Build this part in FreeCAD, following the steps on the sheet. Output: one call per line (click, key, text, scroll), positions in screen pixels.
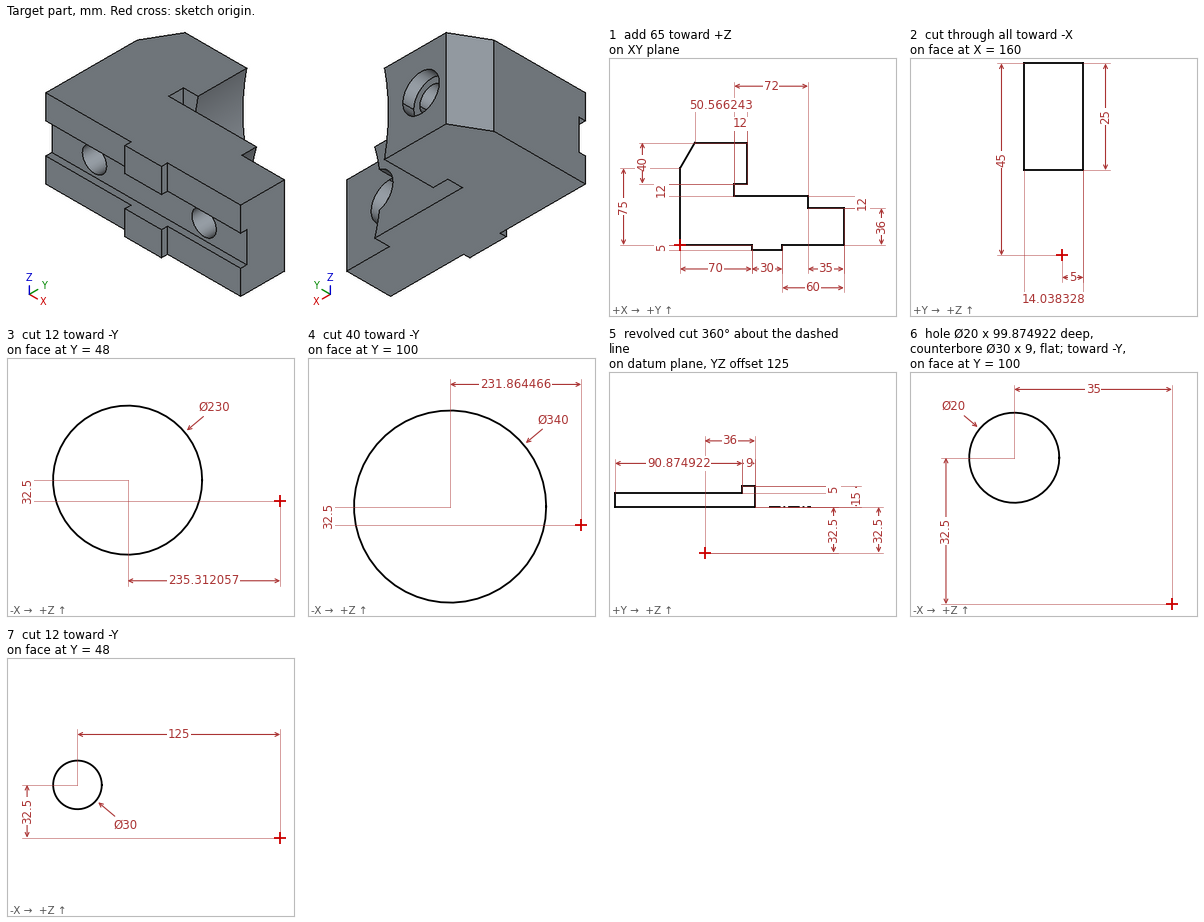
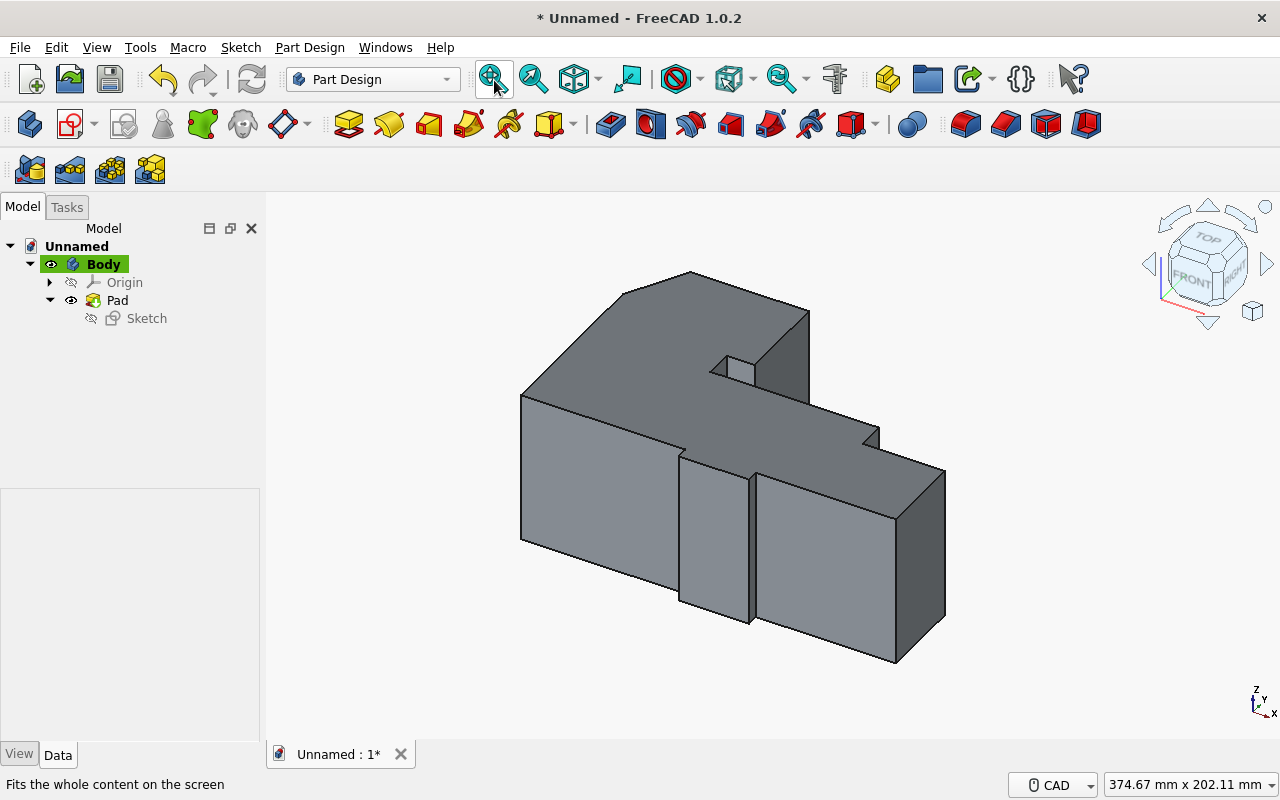
click(921, 546)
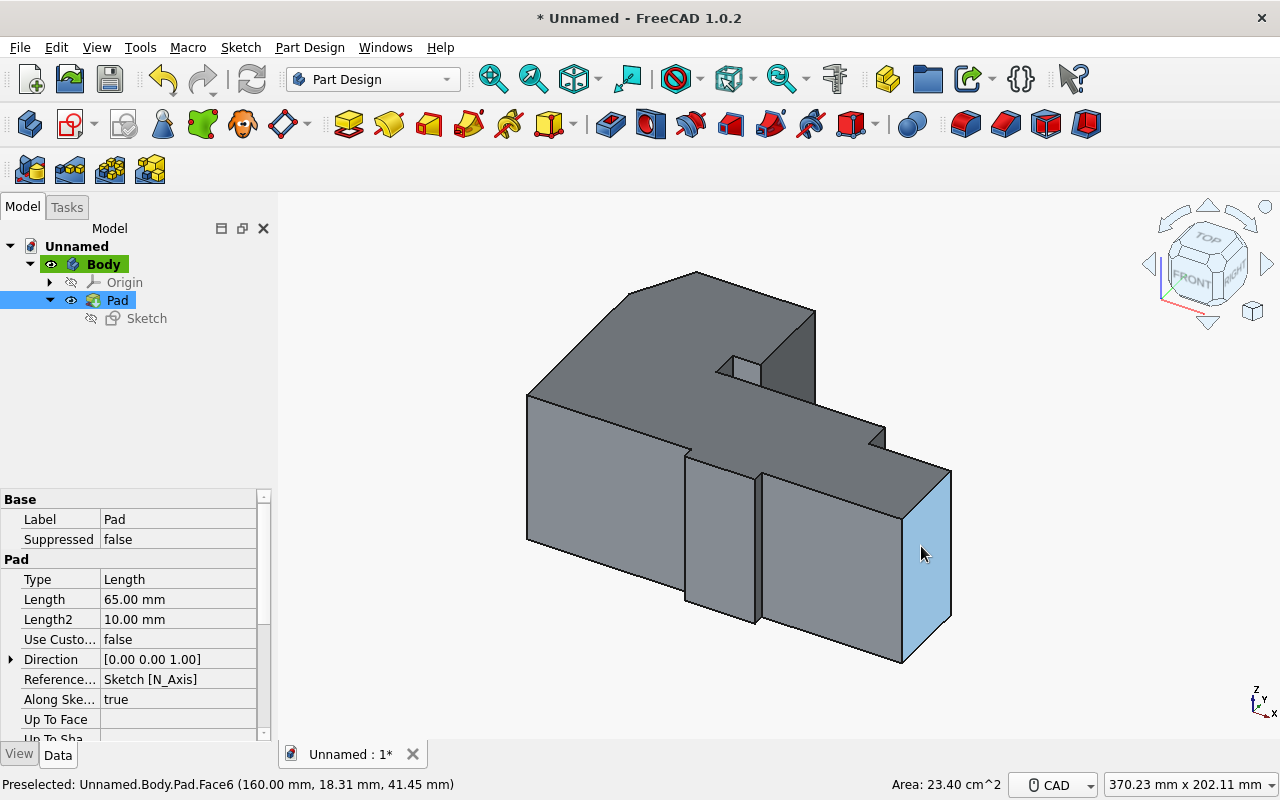
click(70, 124)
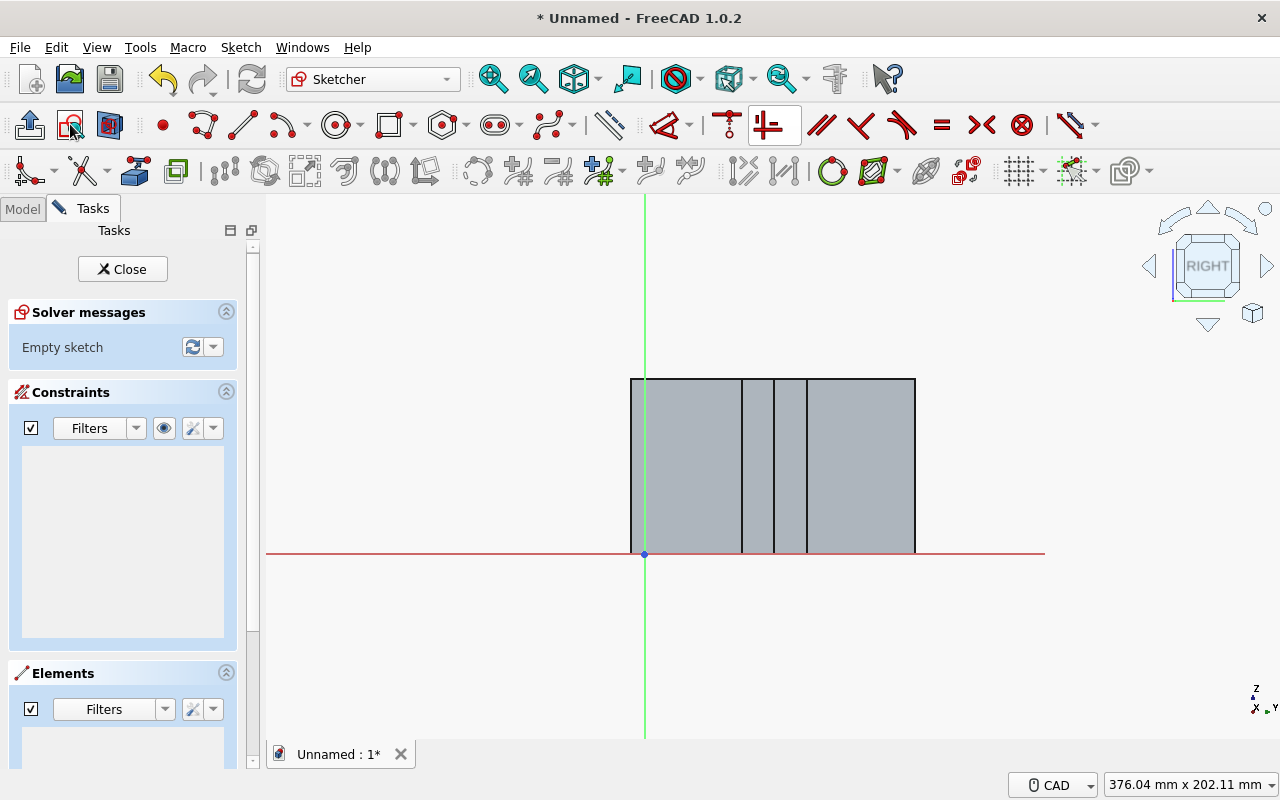
scroll(602, 509, up, 5)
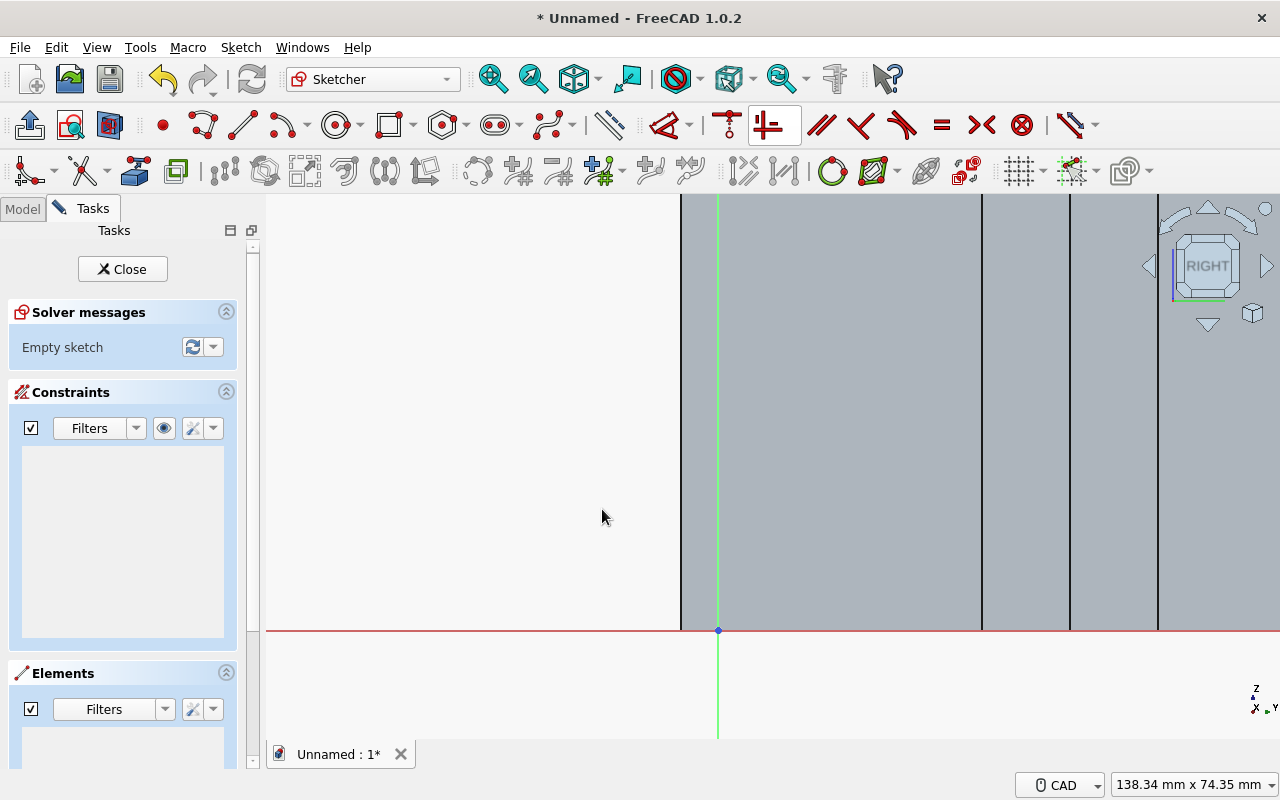
click(390, 126)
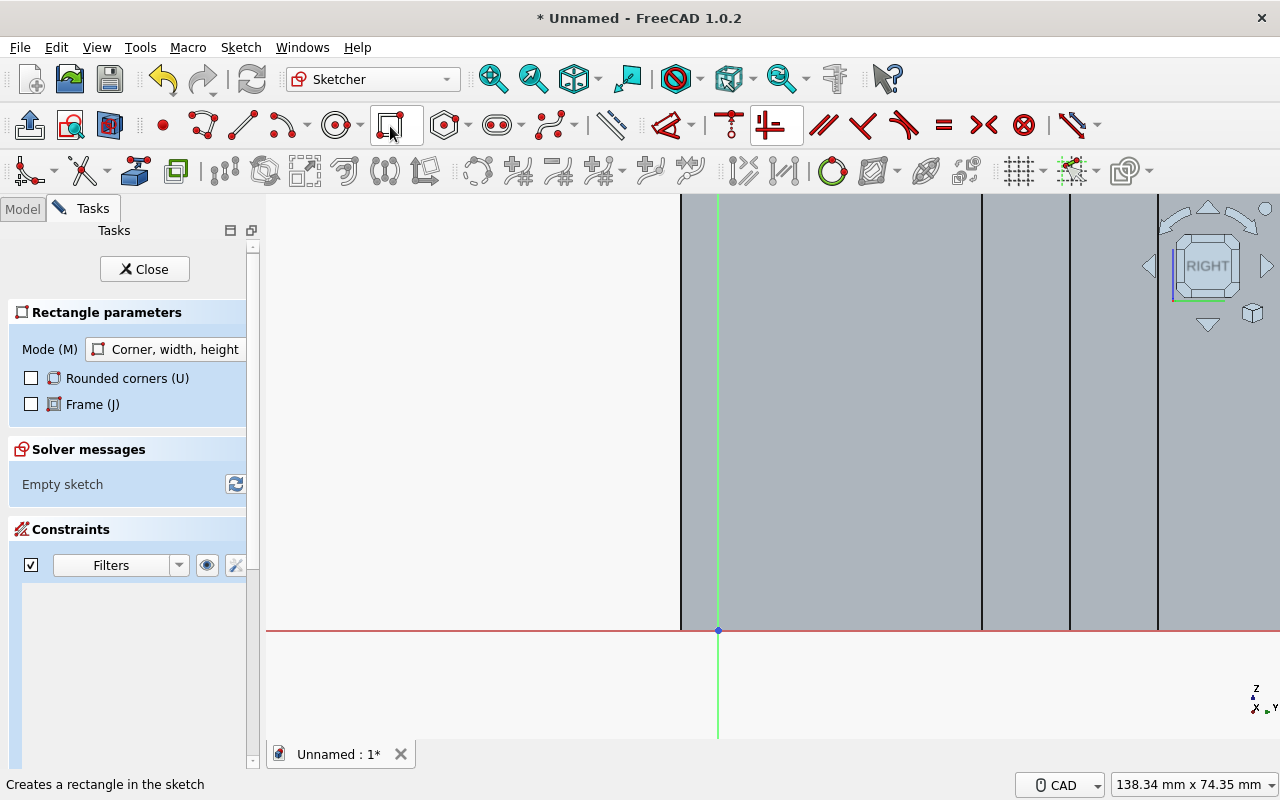
click(652, 301)
move(755, 484)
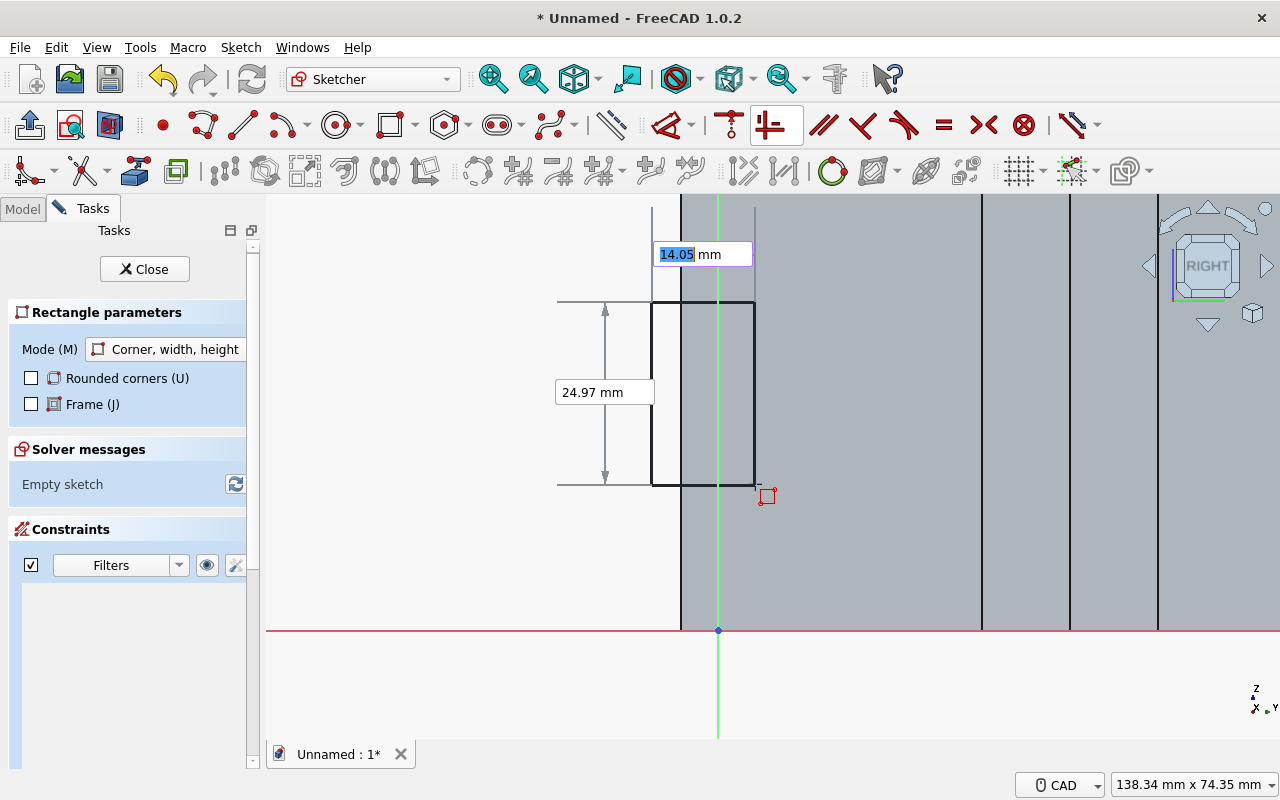
text(14.038328)
key(Tab)
text(25)
key(Return)
key(Escape)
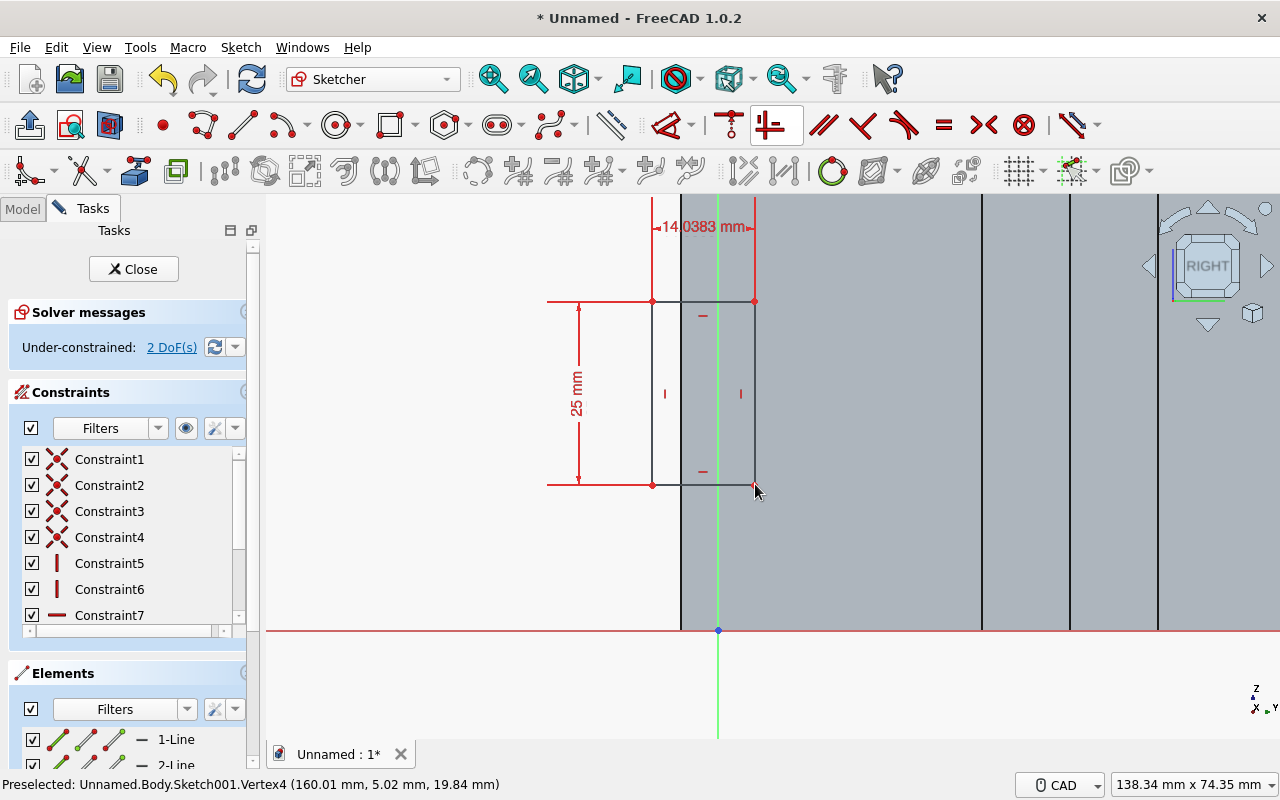
click(666, 126)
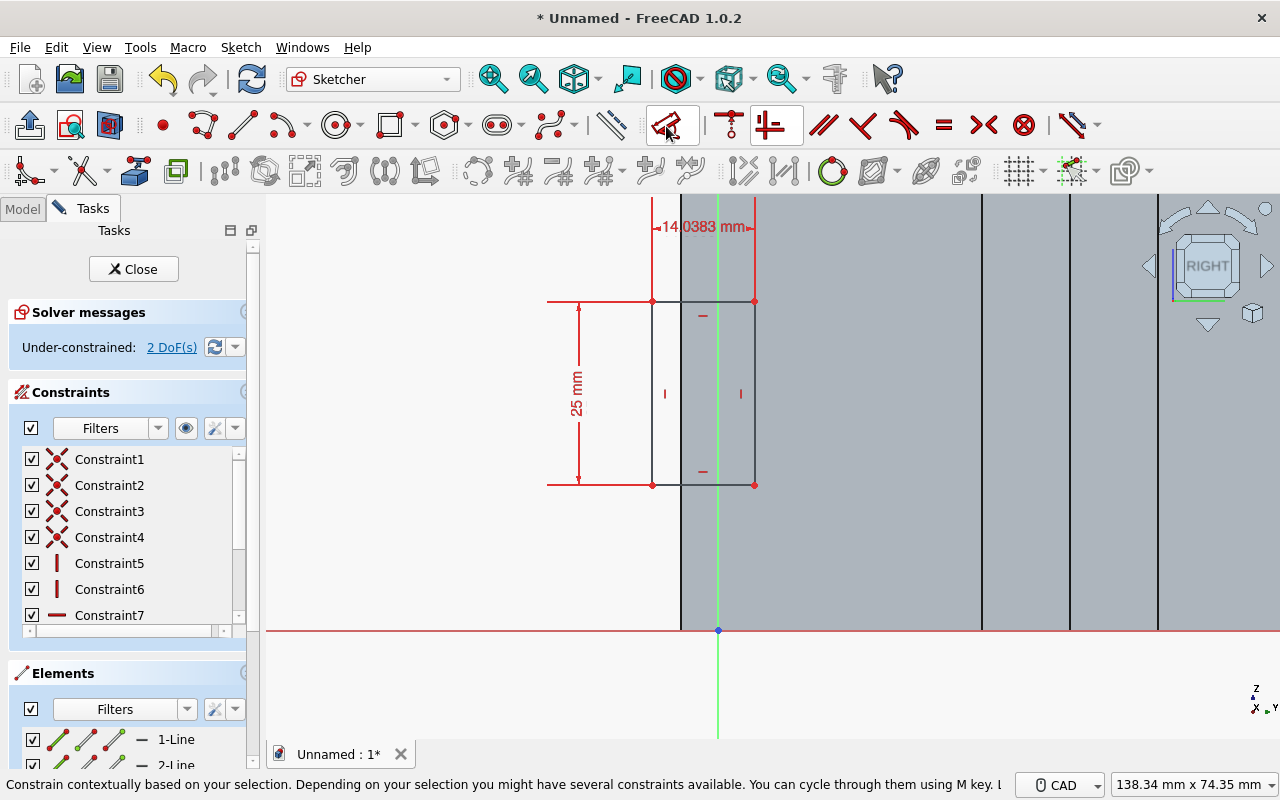
click(755, 485)
click(736, 665)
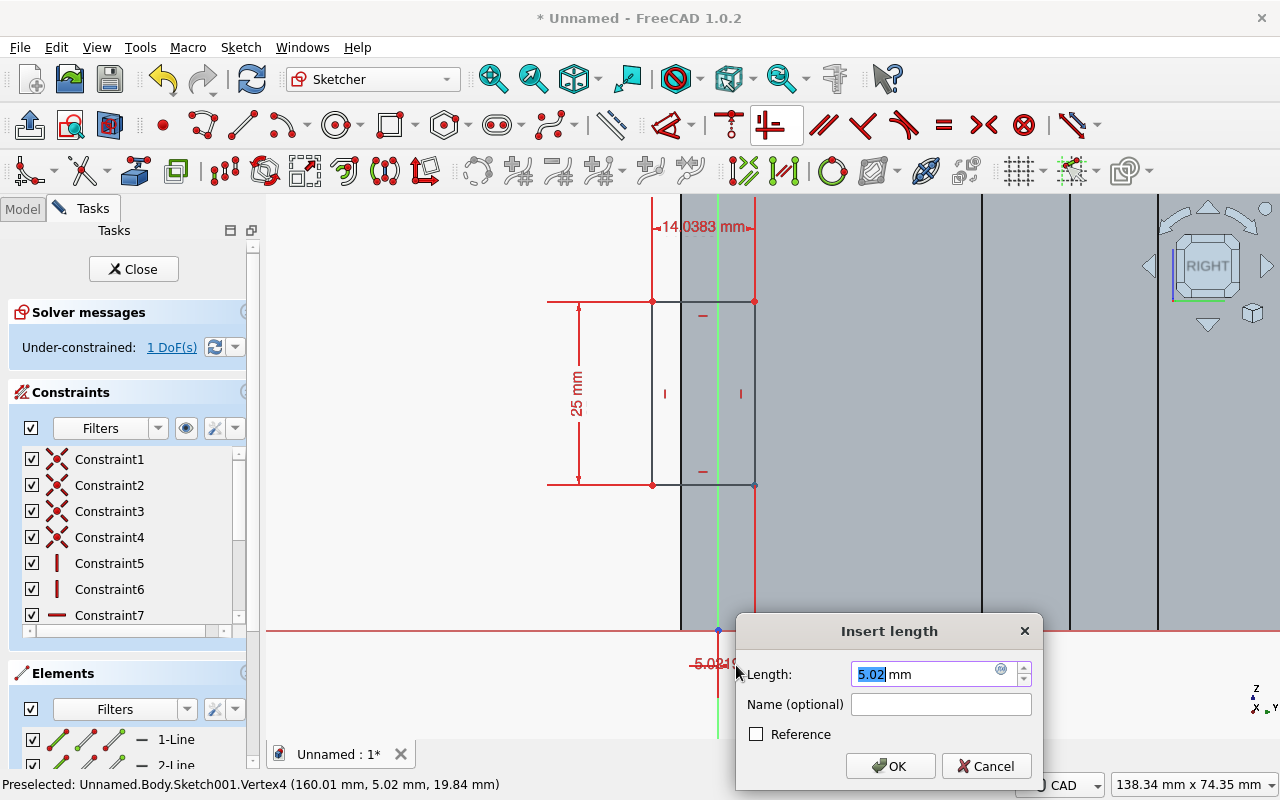
text(5)
key(Return)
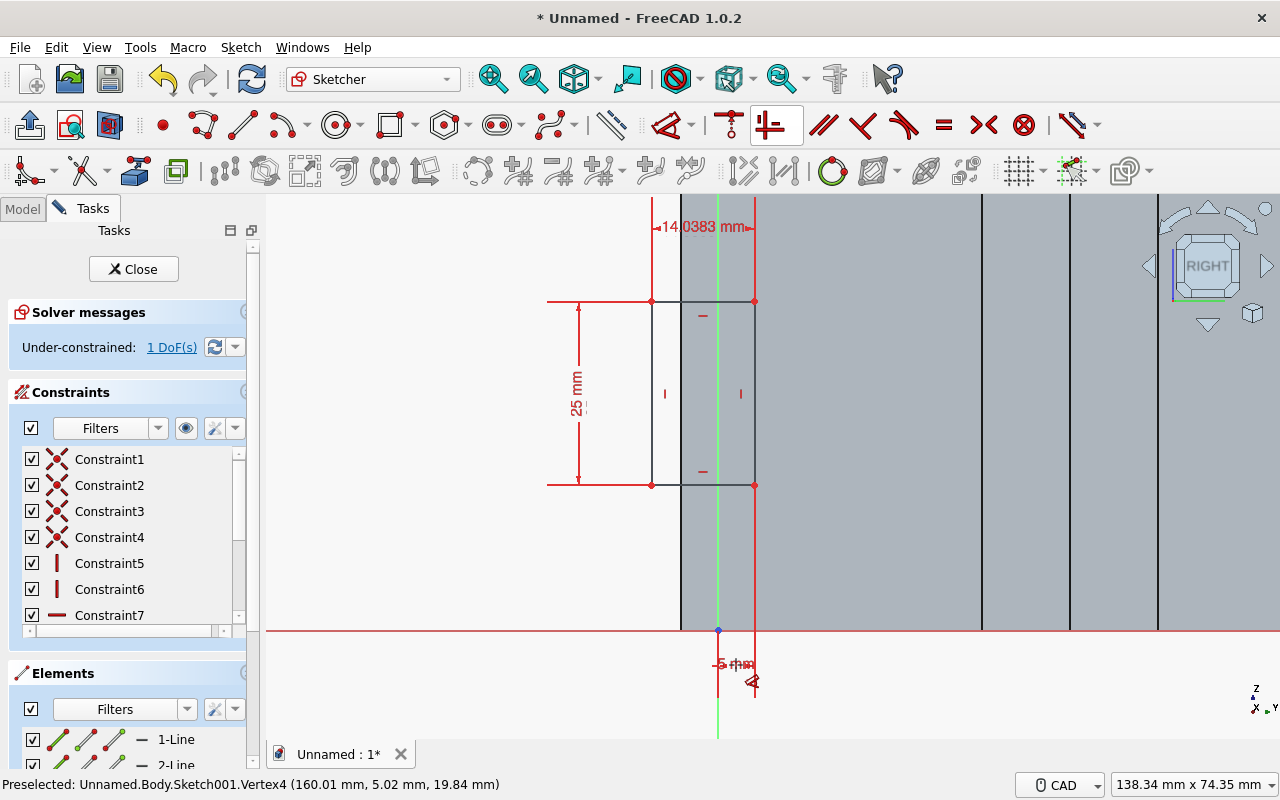
click(652, 302)
click(618, 466)